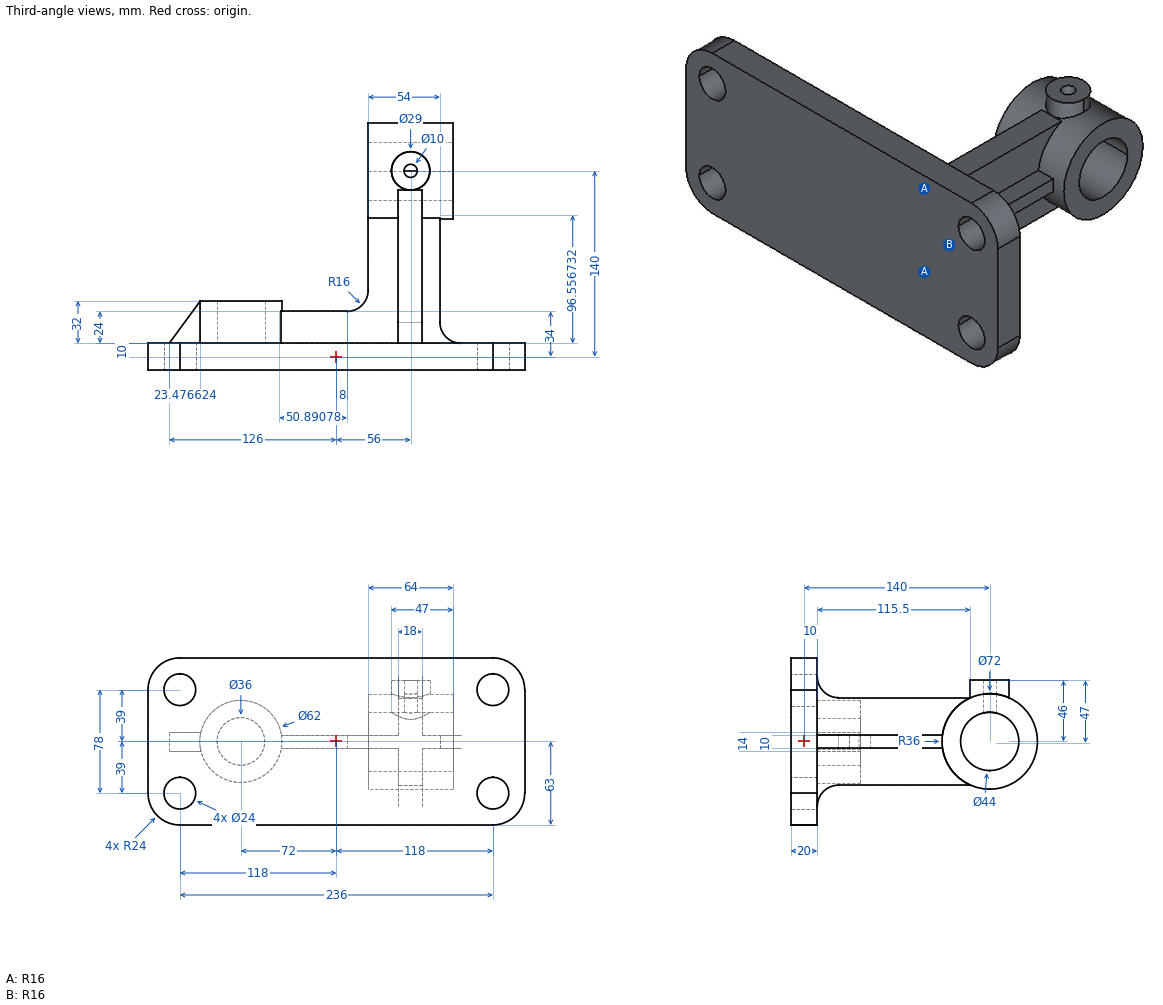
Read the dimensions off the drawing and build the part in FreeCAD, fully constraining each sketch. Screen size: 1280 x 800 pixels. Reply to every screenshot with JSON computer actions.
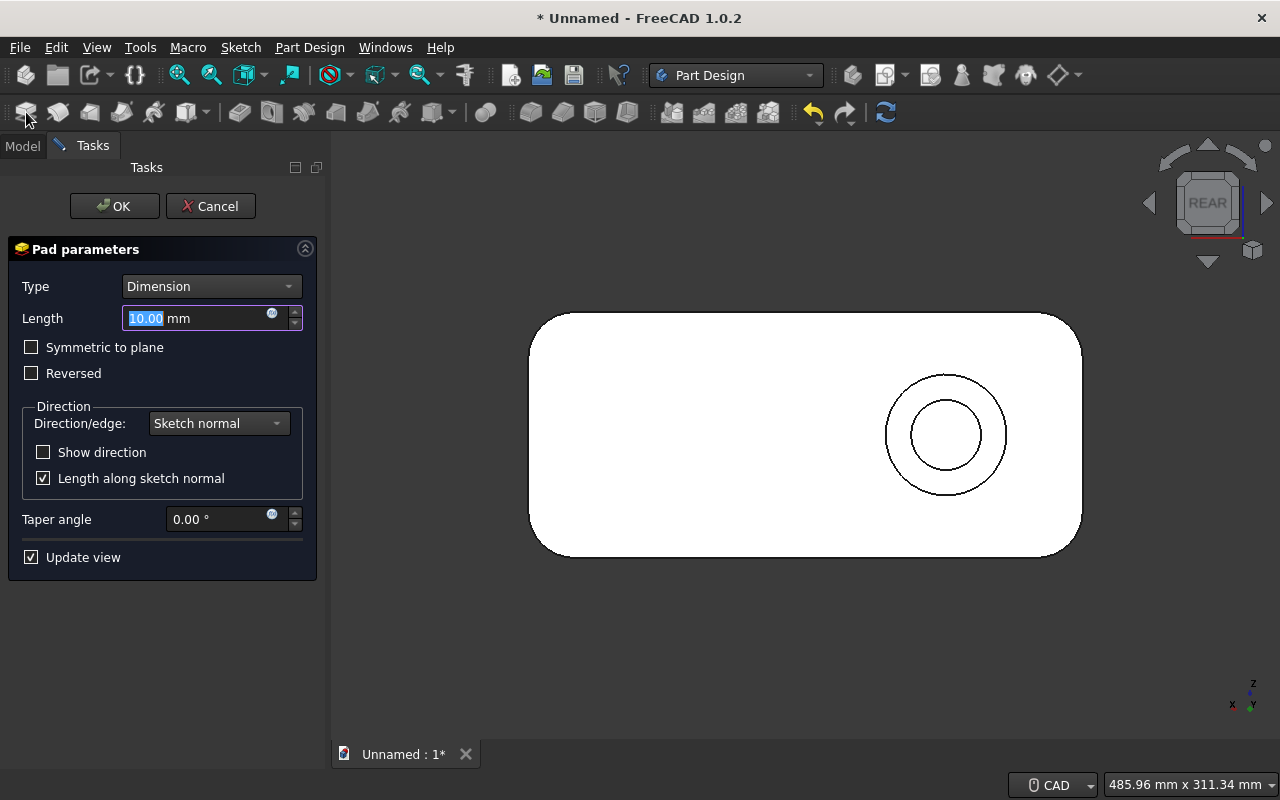
{"action": "type", "text": "32"}
{"action": "key", "text": "Tab"}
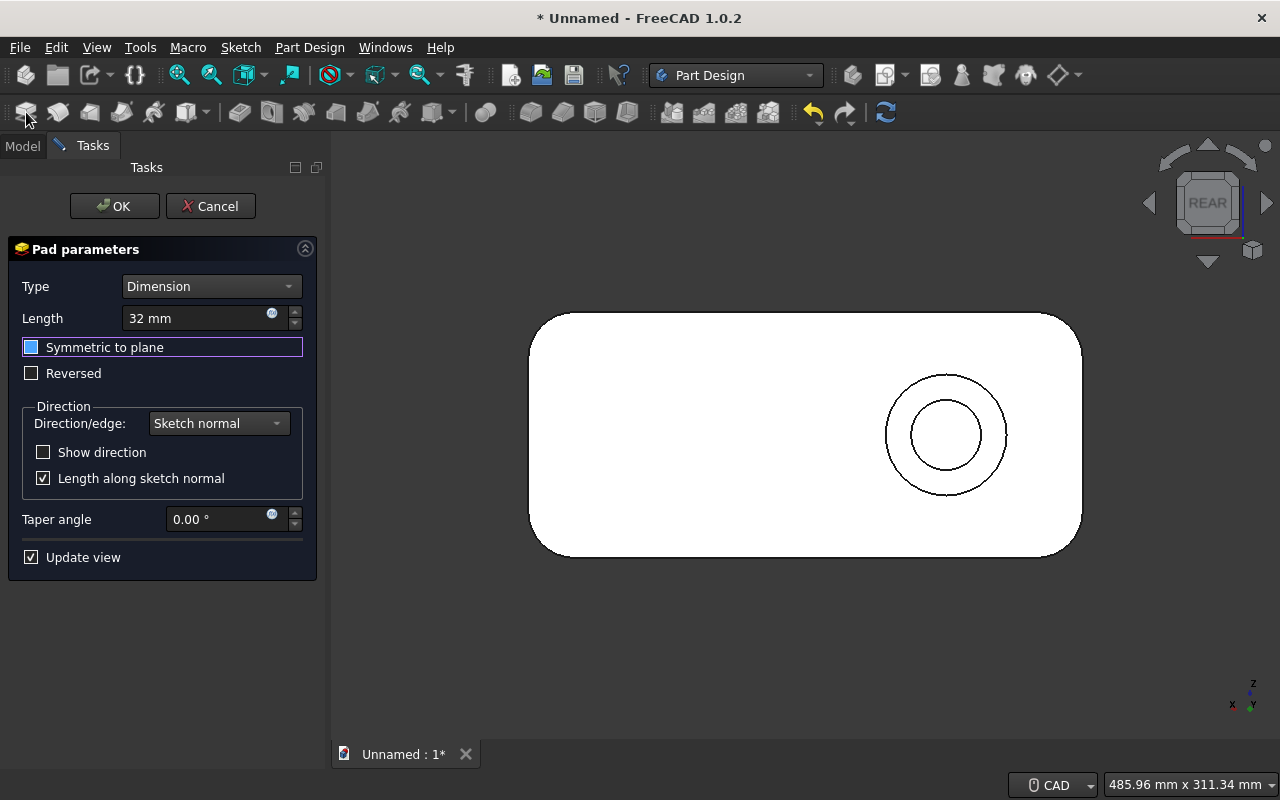
{"action": "left_click", "coordinate": [115, 206]}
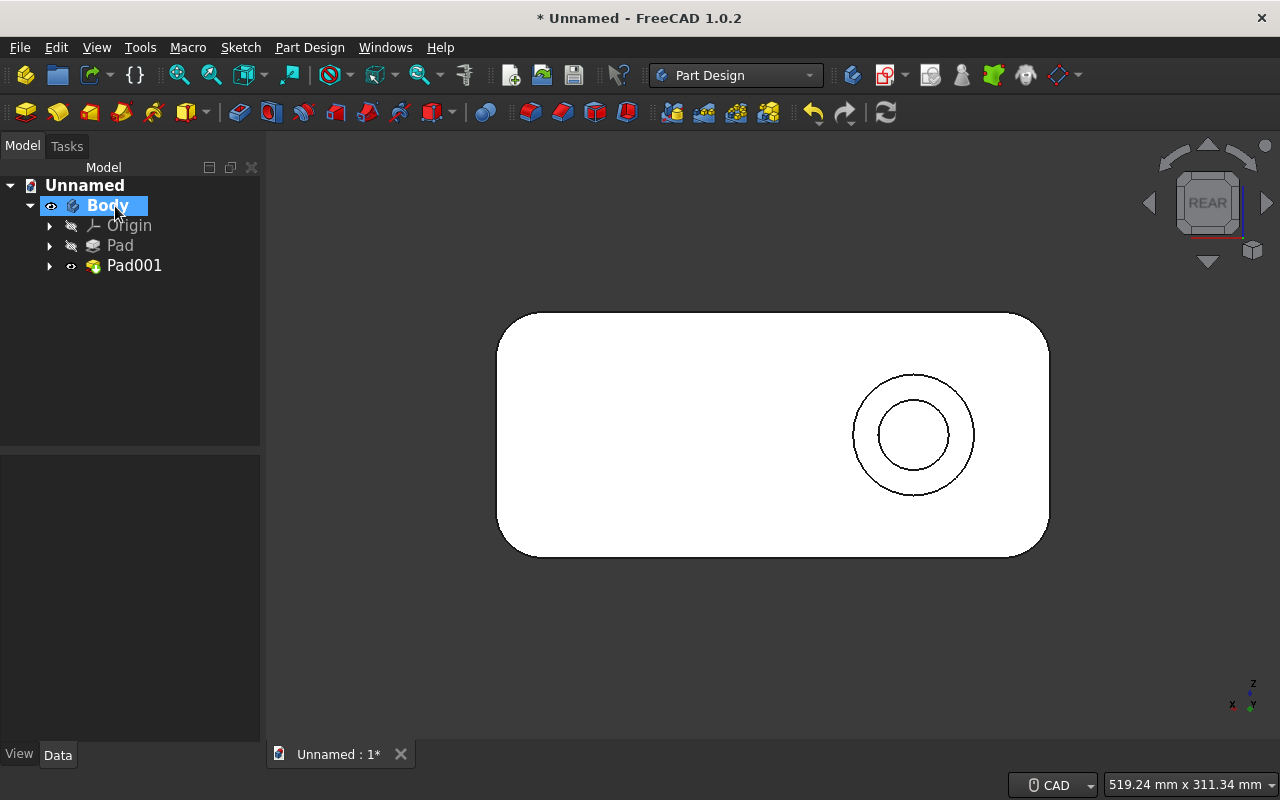
{"action": "left_click", "coordinate": [886, 76]}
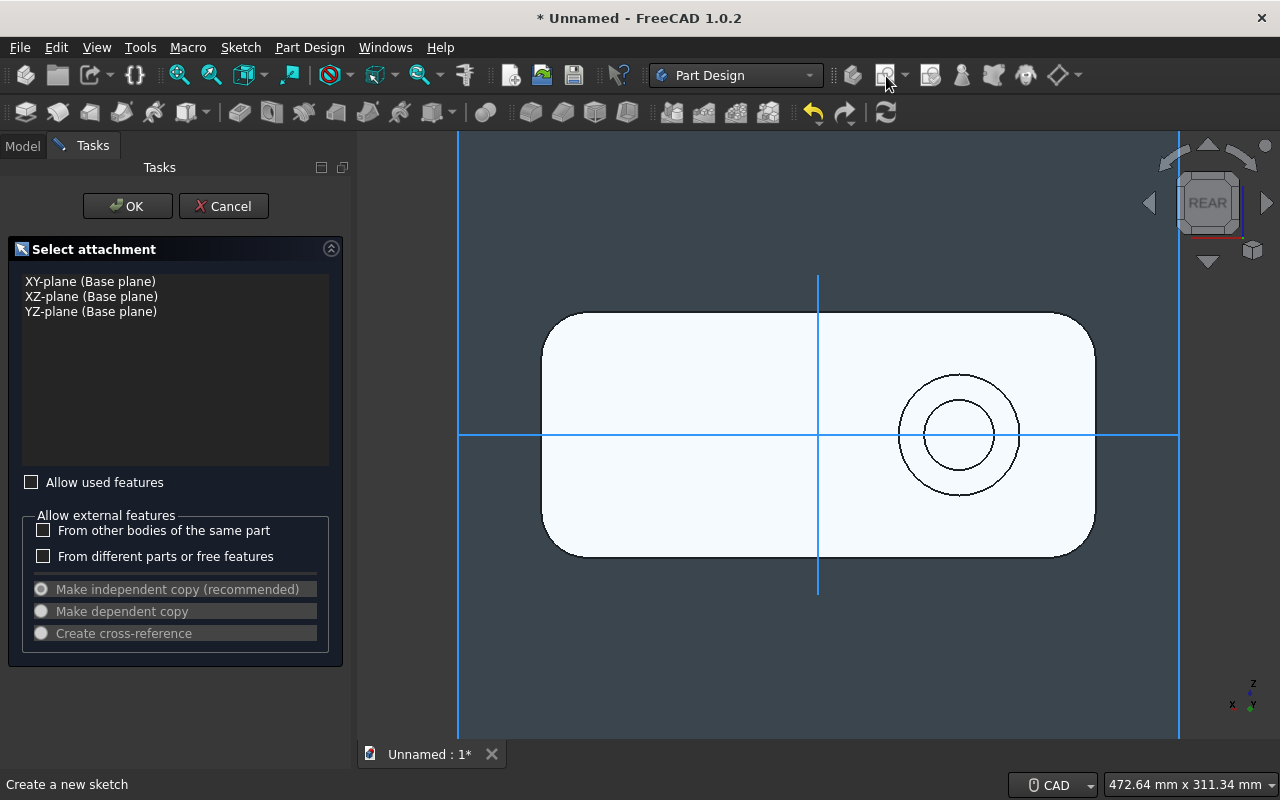
{"action": "left_click", "coordinate": [82, 282]}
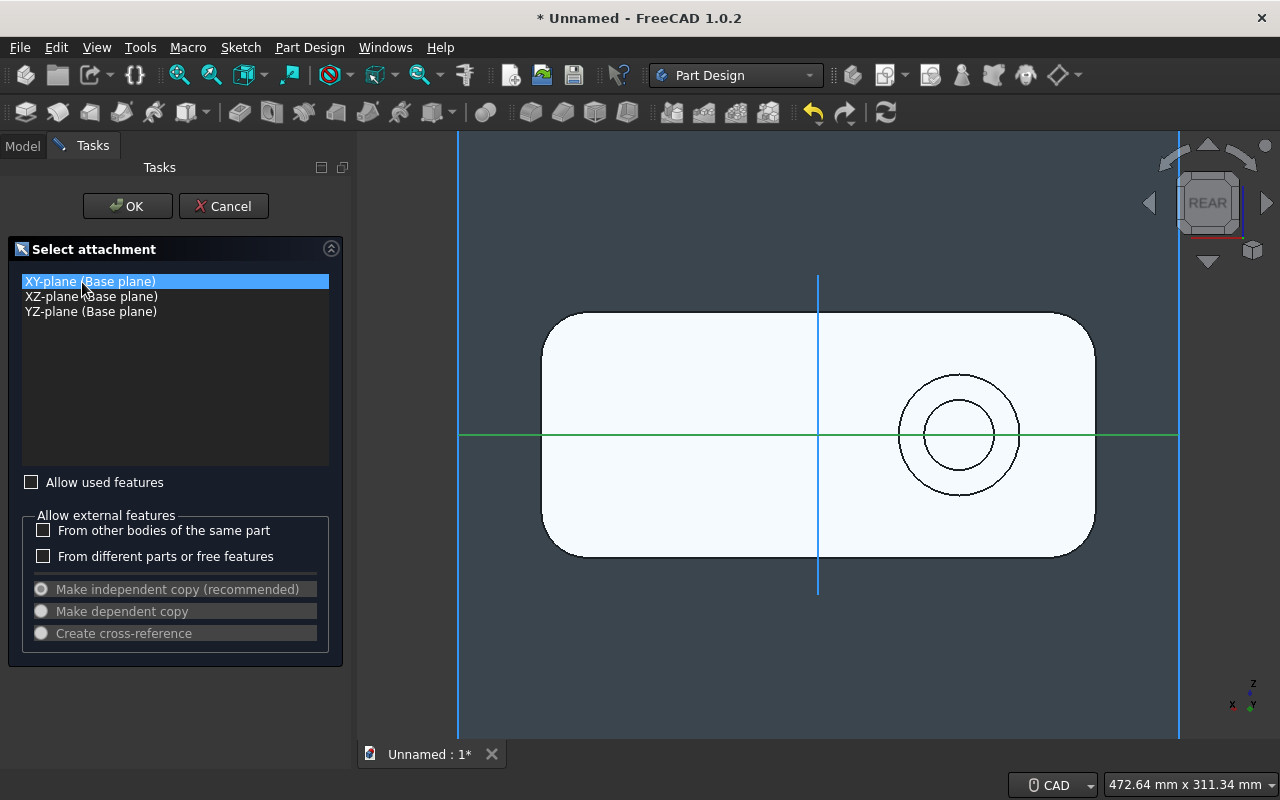
{"action": "left_click", "coordinate": [128, 206]}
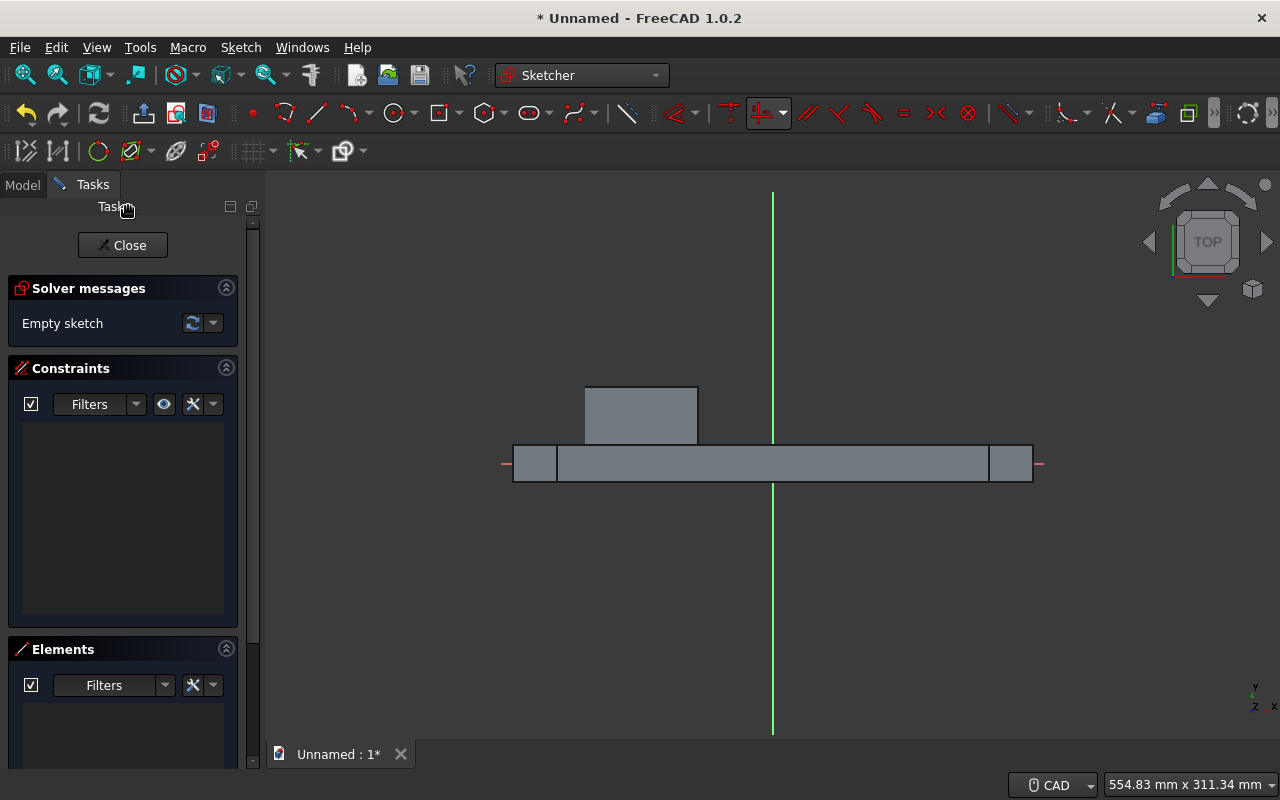
{"action": "left_click", "coordinate": [208, 114]}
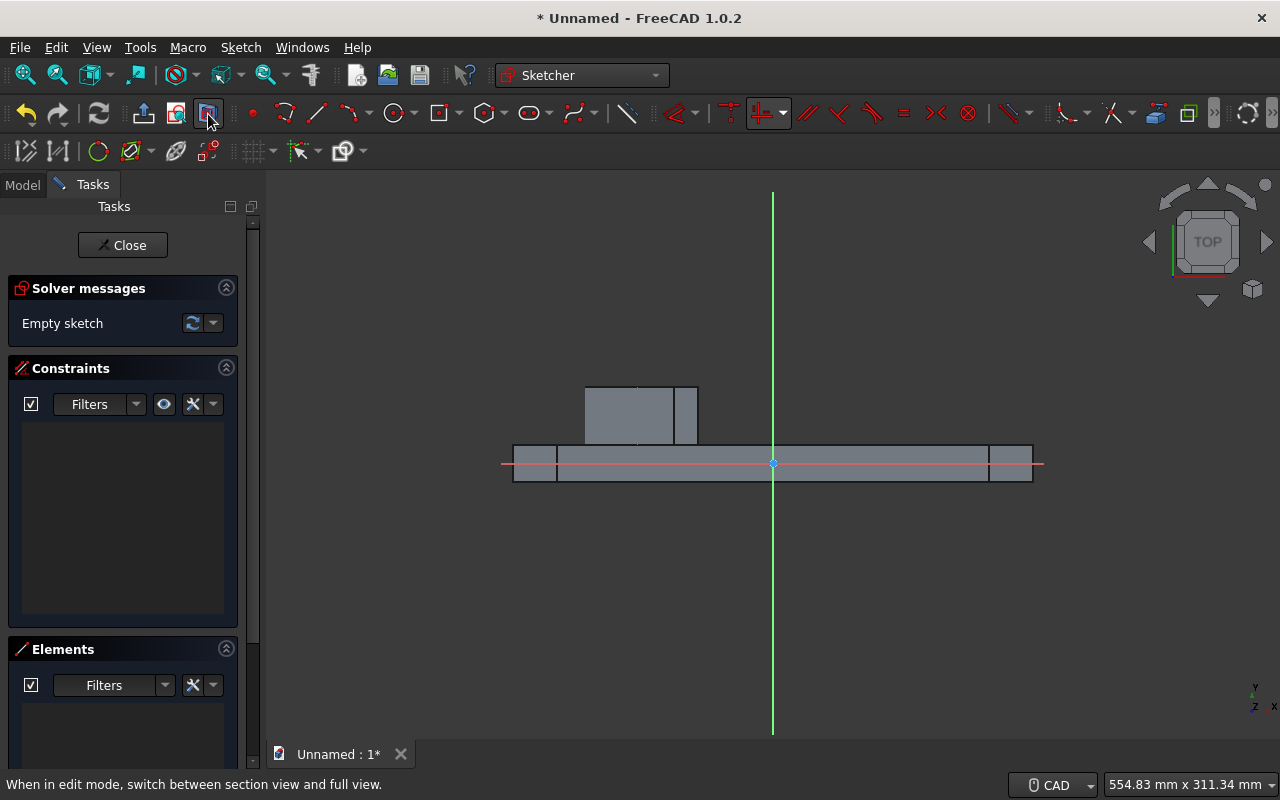
{"action": "scroll", "coordinate": [536, 409], "scroll_direction": "up", "scroll_amount": 9}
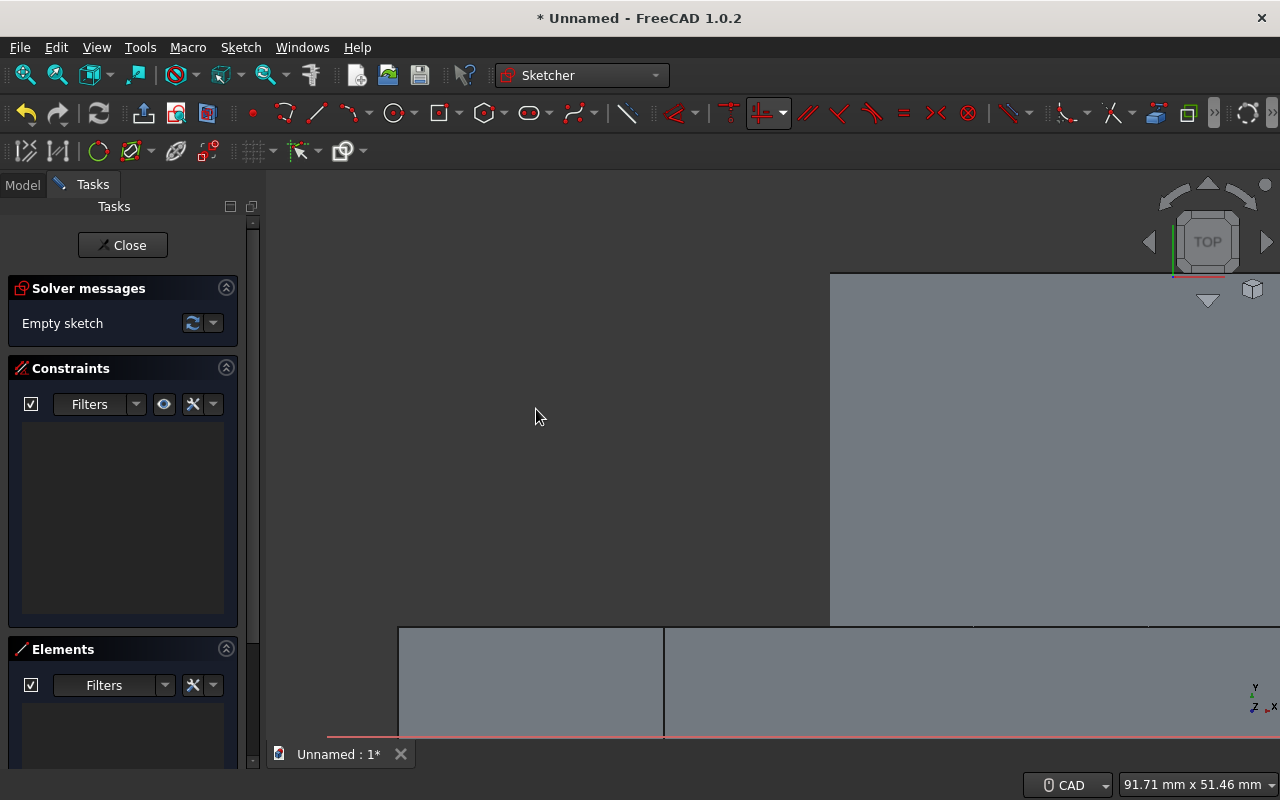
{"action": "left_click", "coordinate": [286, 114]}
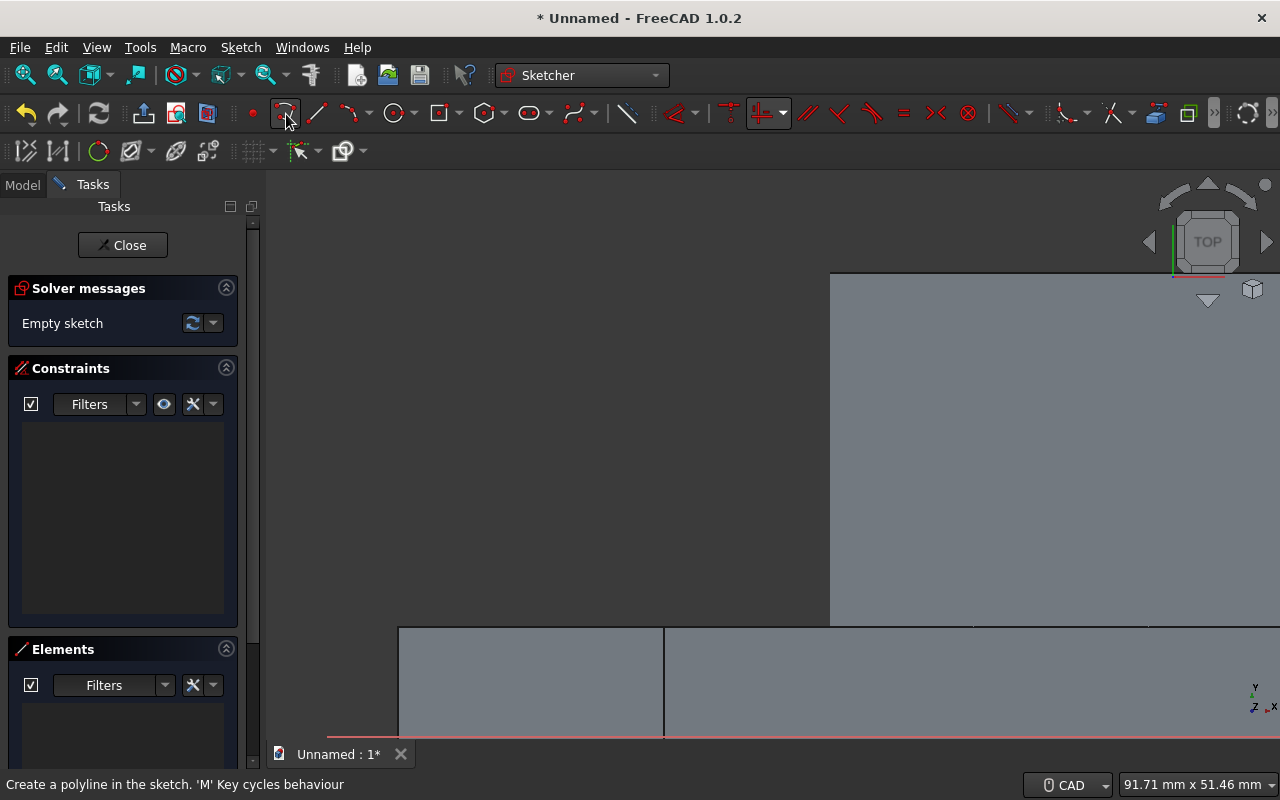
{"action": "left_click", "coordinate": [835, 627]}
{"action": "left_click", "coordinate": [835, 273]}
{"action": "left_click", "coordinate": [575, 627]}
{"action": "left_click", "coordinate": [835, 628]}
{"action": "key", "text": "Escape"}
{"action": "key", "text": "Escape"}